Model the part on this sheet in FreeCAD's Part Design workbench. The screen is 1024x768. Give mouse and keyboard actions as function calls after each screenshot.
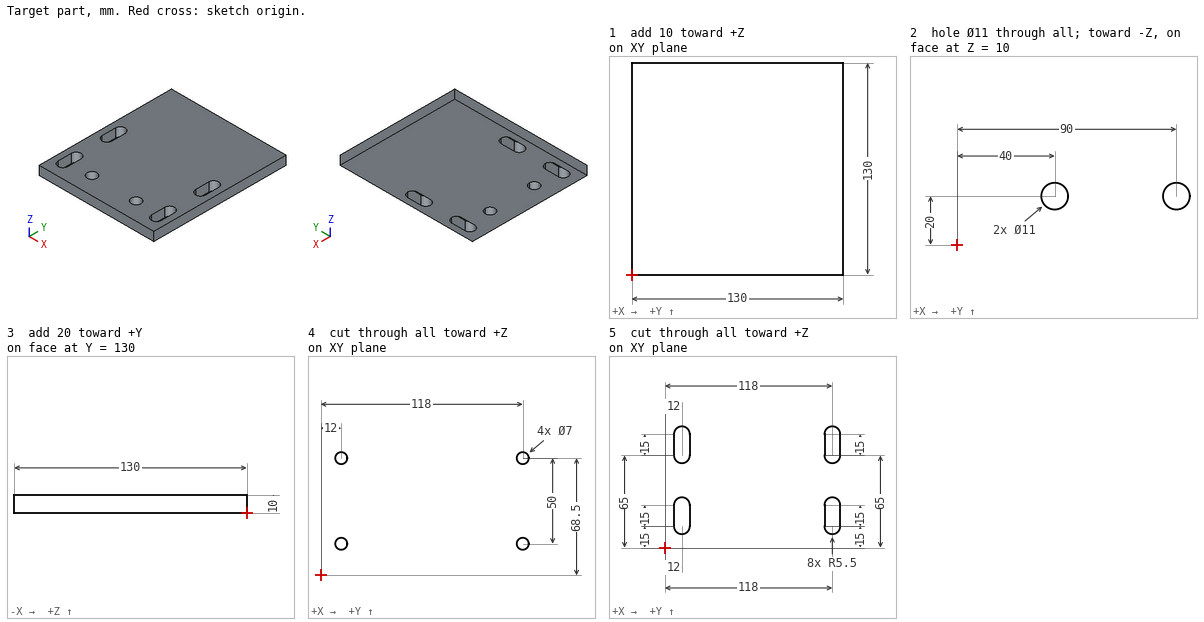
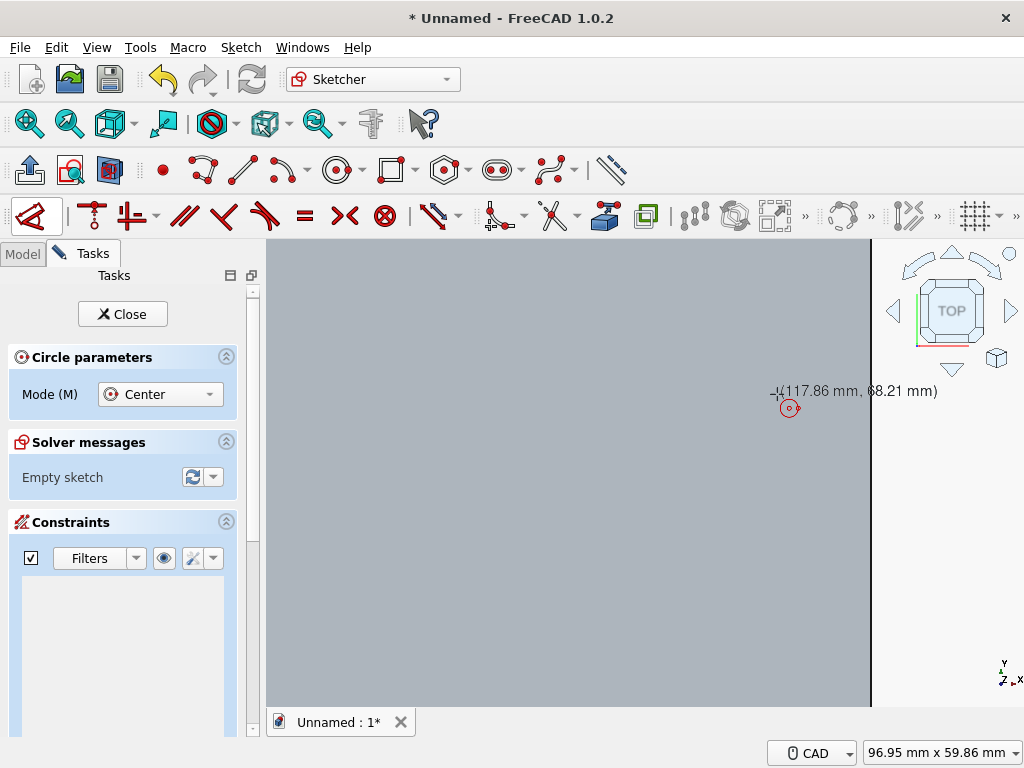
click(777, 394)
click(797, 374)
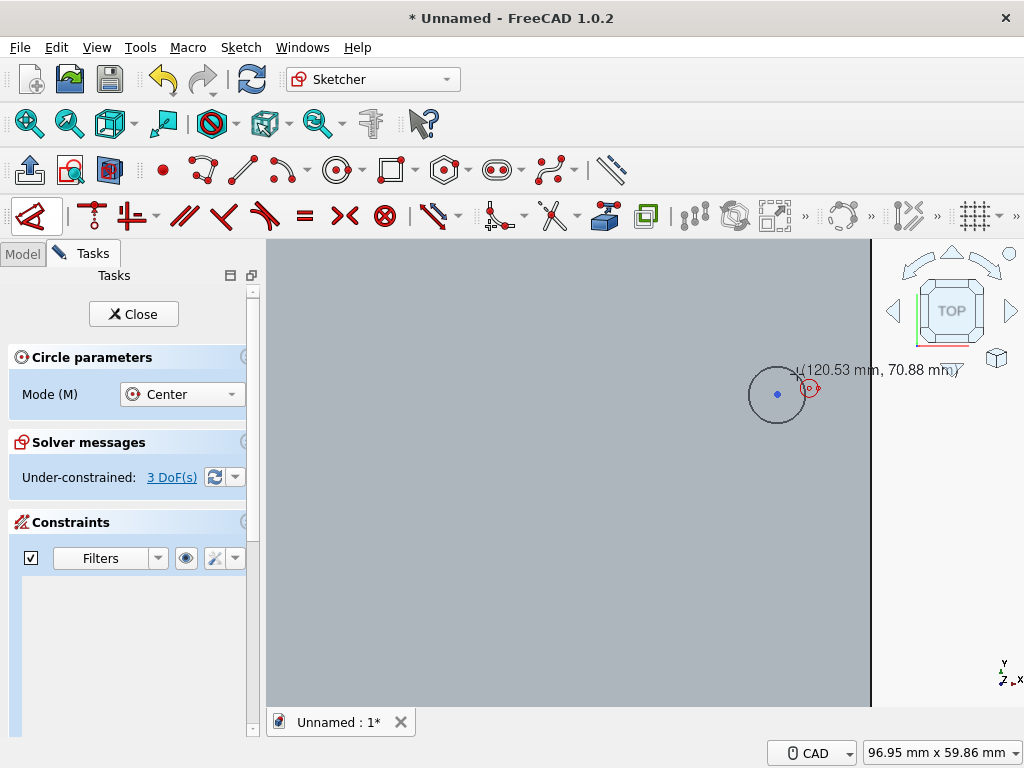
scroll(778, 330, down, 4)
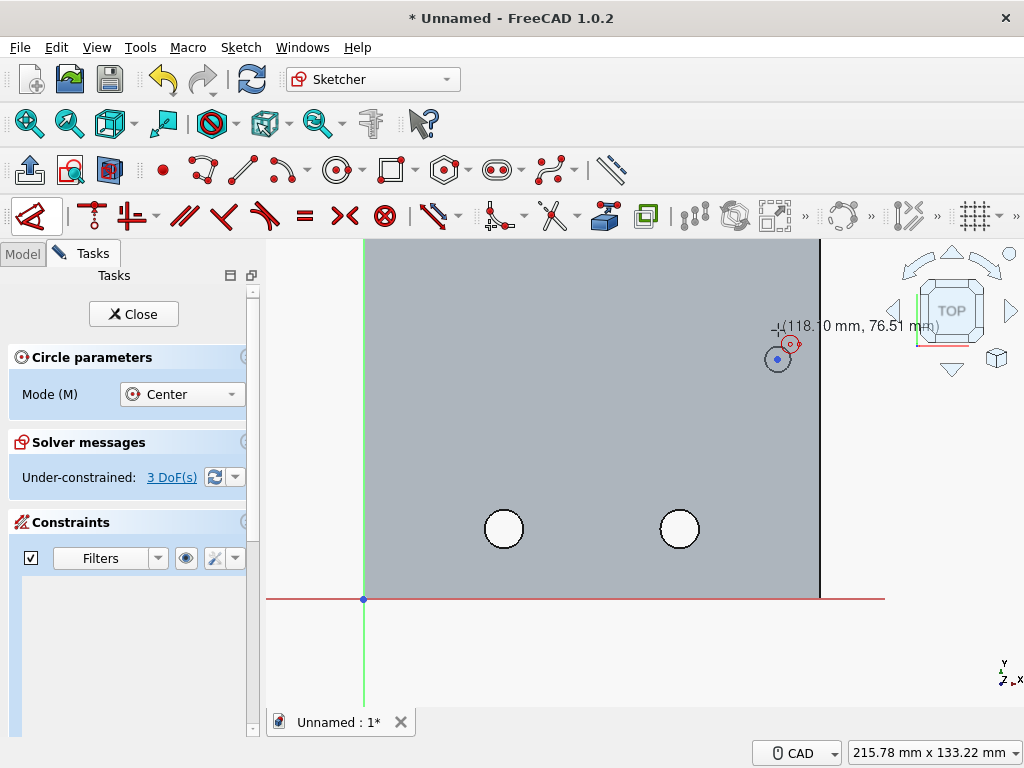
scroll(778, 534, up, 4)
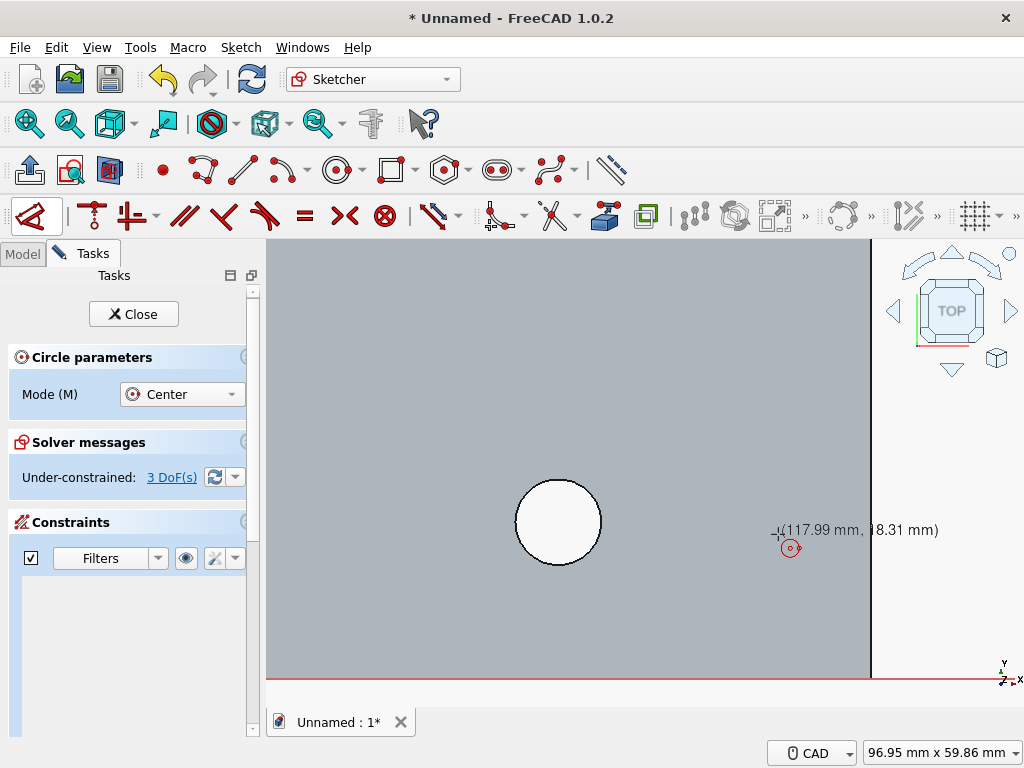
click(777, 534)
click(797, 515)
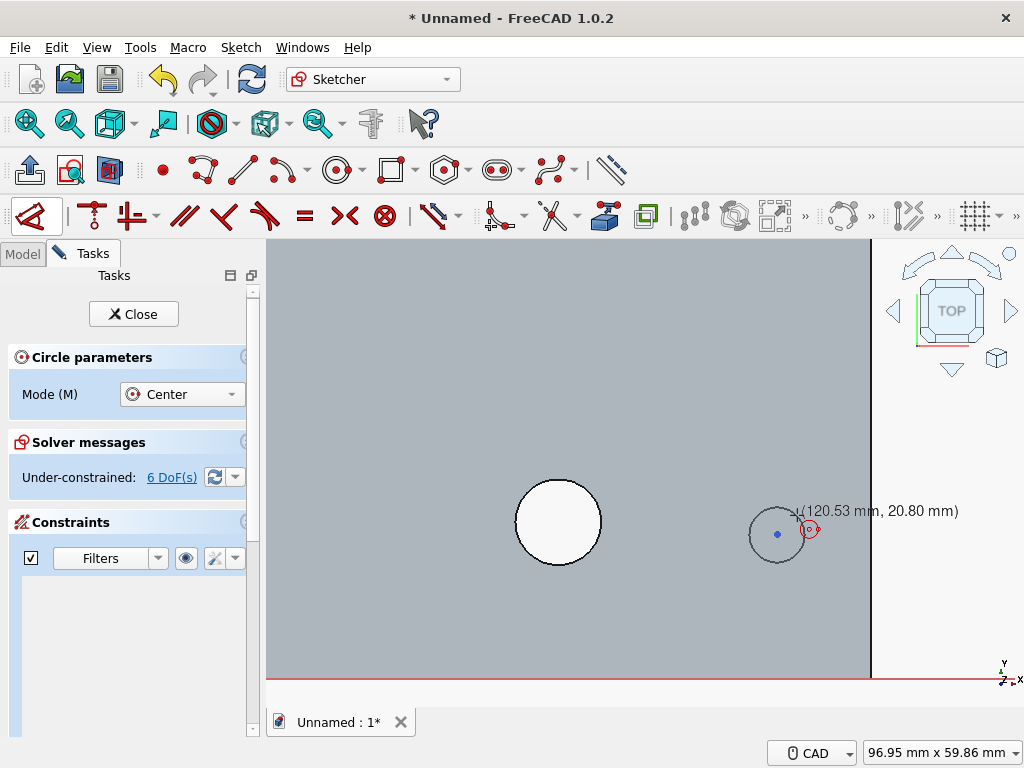
scroll(778, 535, down, 4)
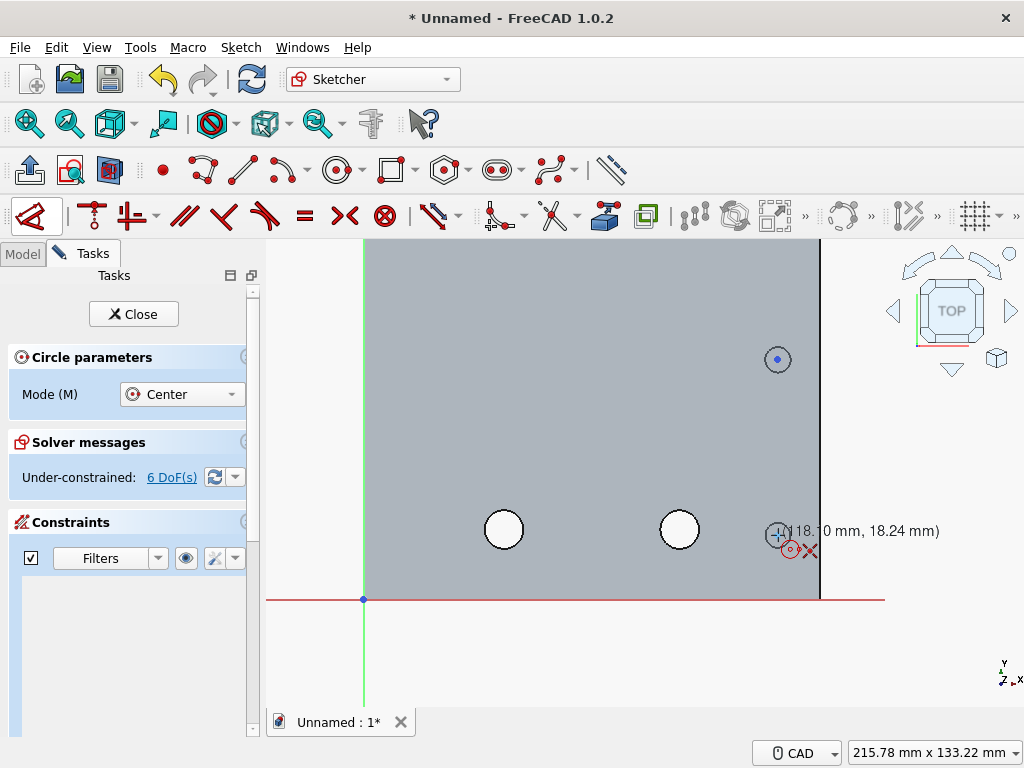
scroll(406, 359, up, 4)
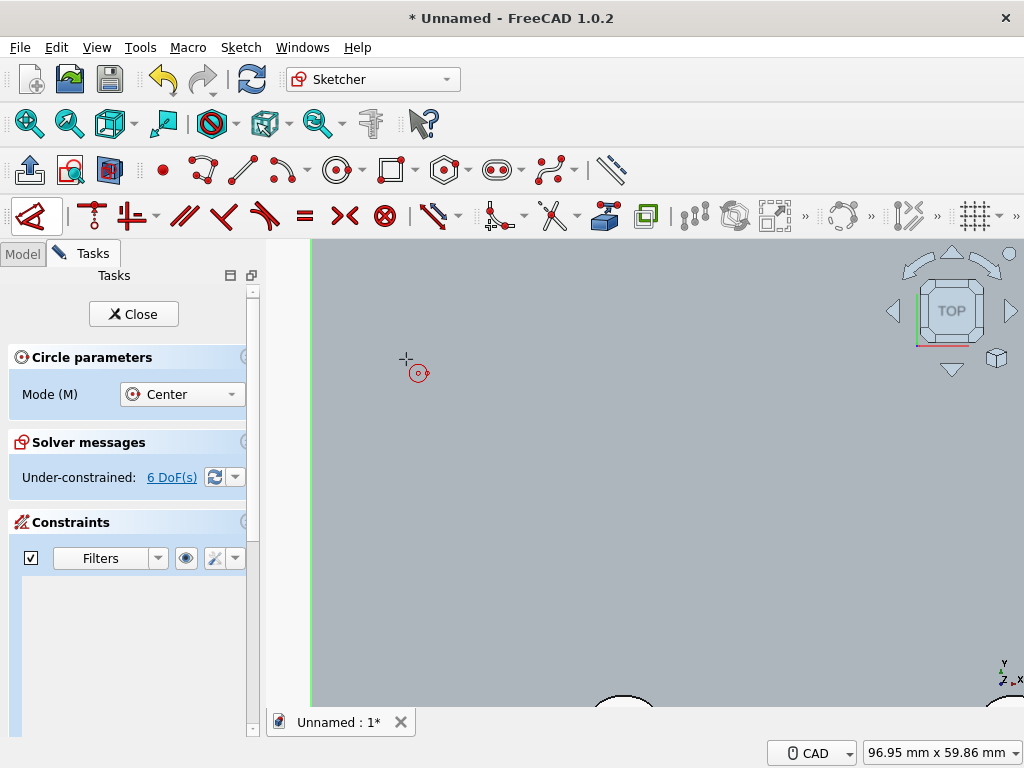
click(405, 359)
click(424, 340)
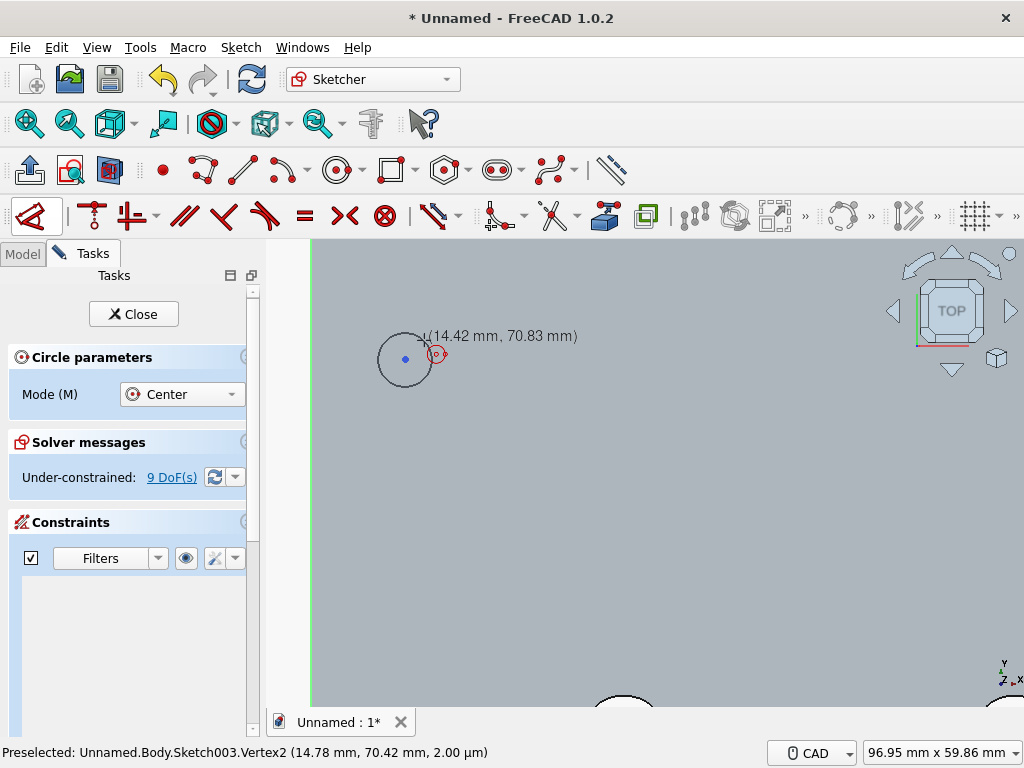
scroll(405, 359, down, 4)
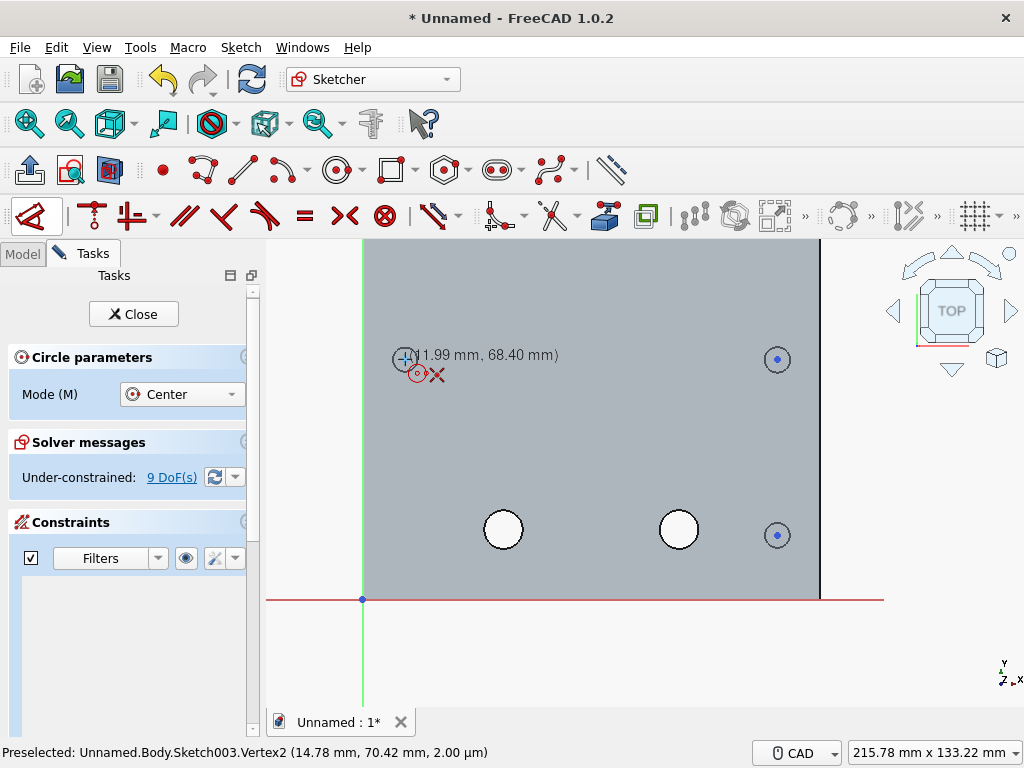
scroll(405, 535, up, 4)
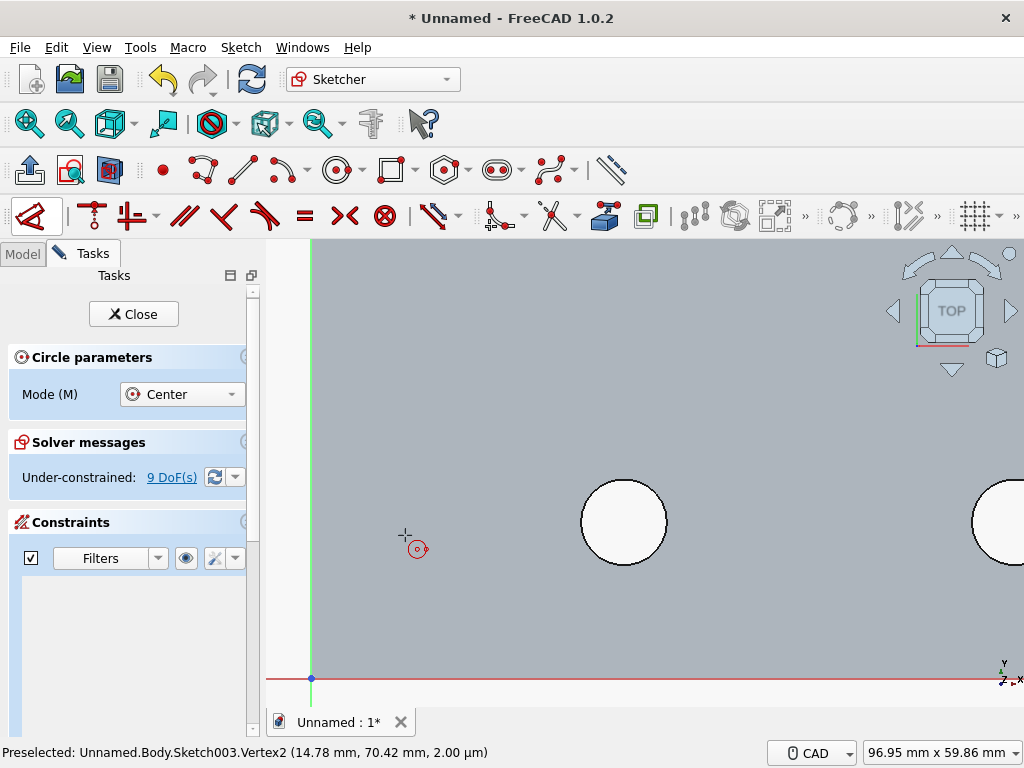
click(405, 534)
click(424, 515)
key(Escape)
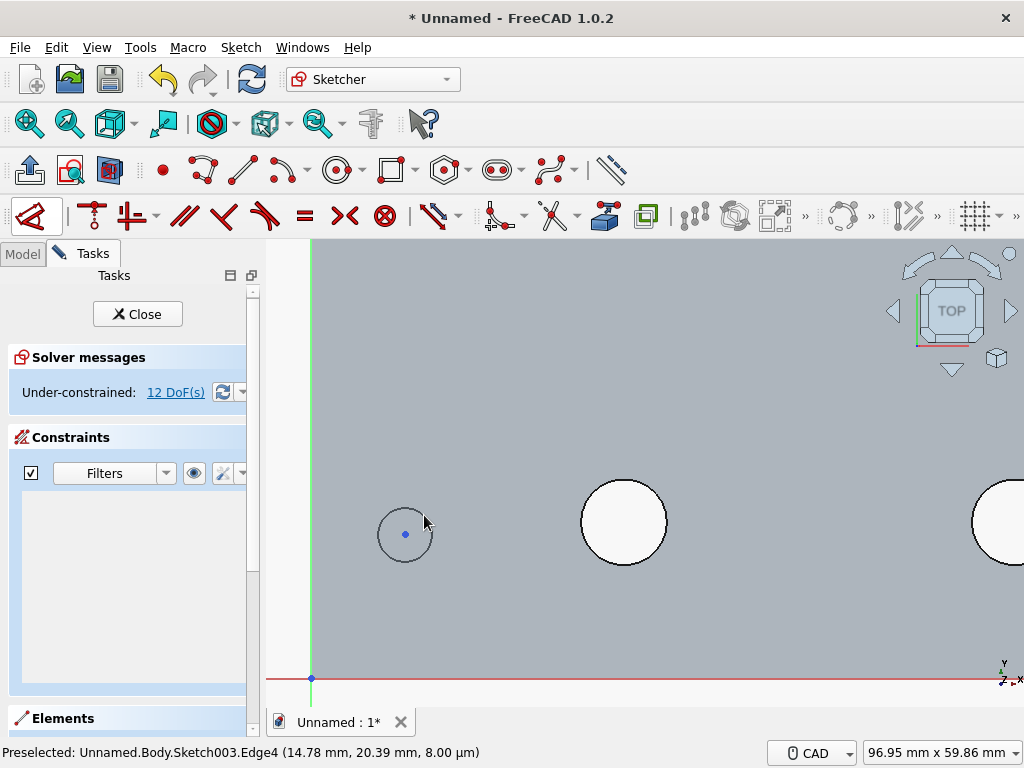
scroll(405, 535, down, 4)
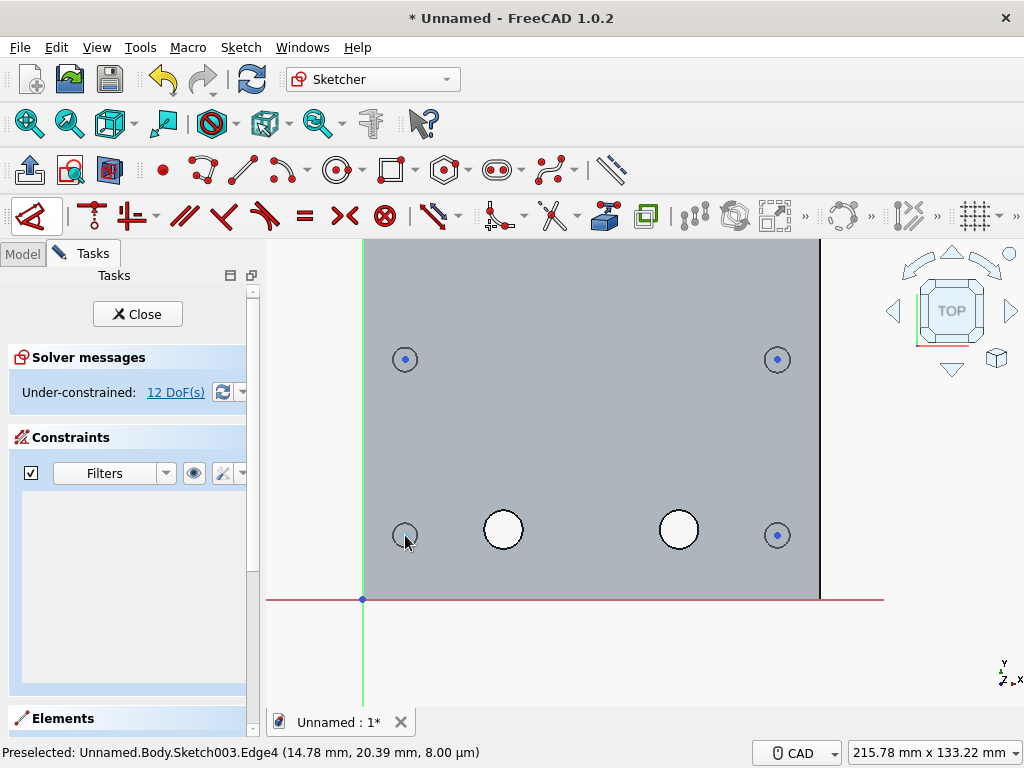
click(786, 351)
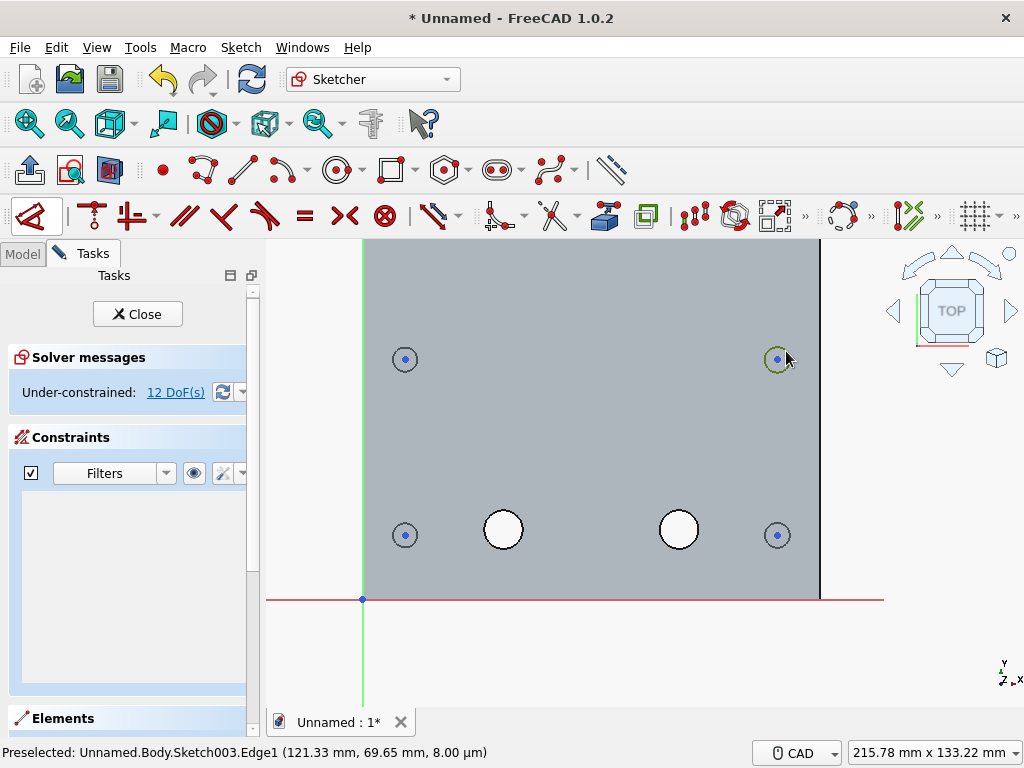
click(786, 527)